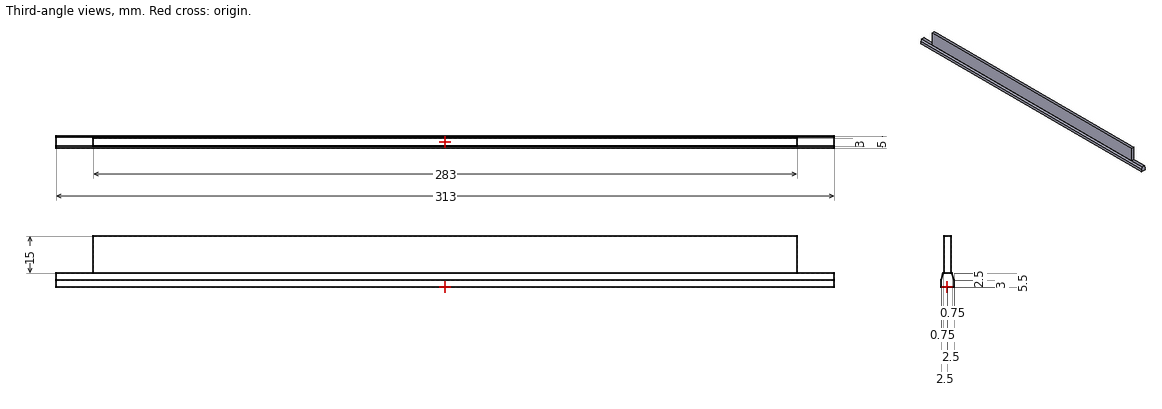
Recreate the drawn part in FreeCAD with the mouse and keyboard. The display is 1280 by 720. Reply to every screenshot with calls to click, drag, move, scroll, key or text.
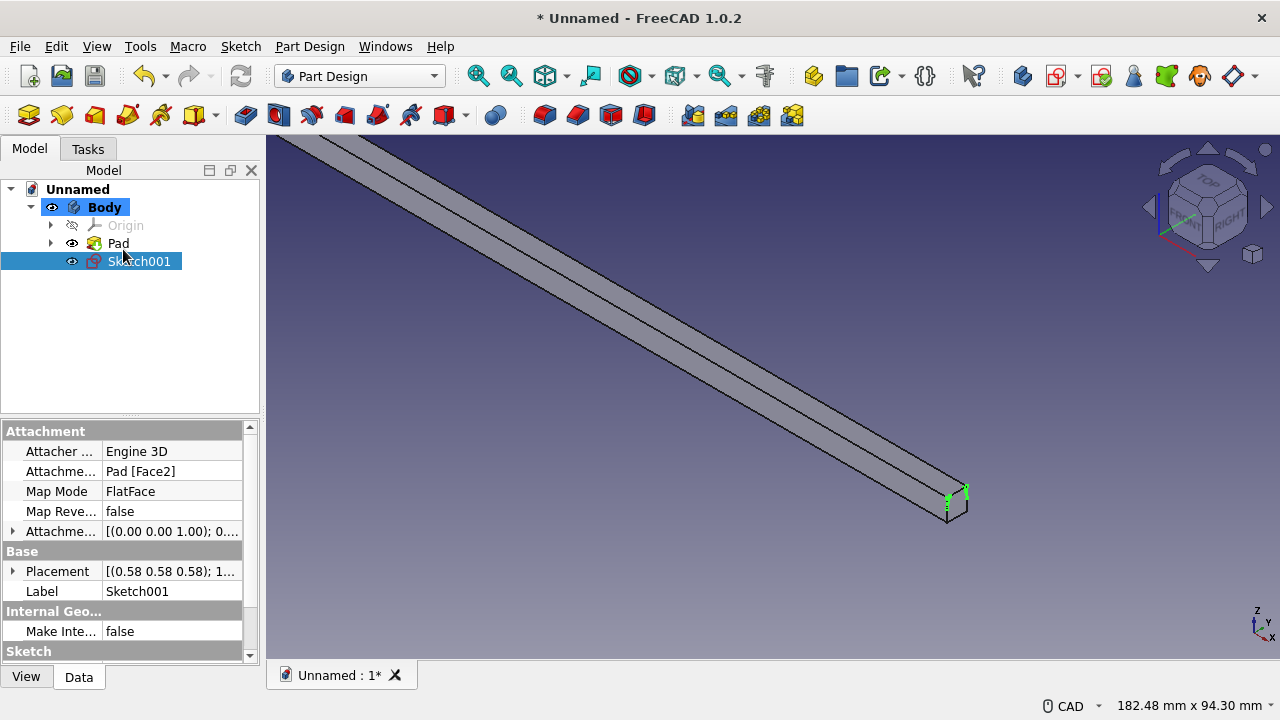
click(246, 116)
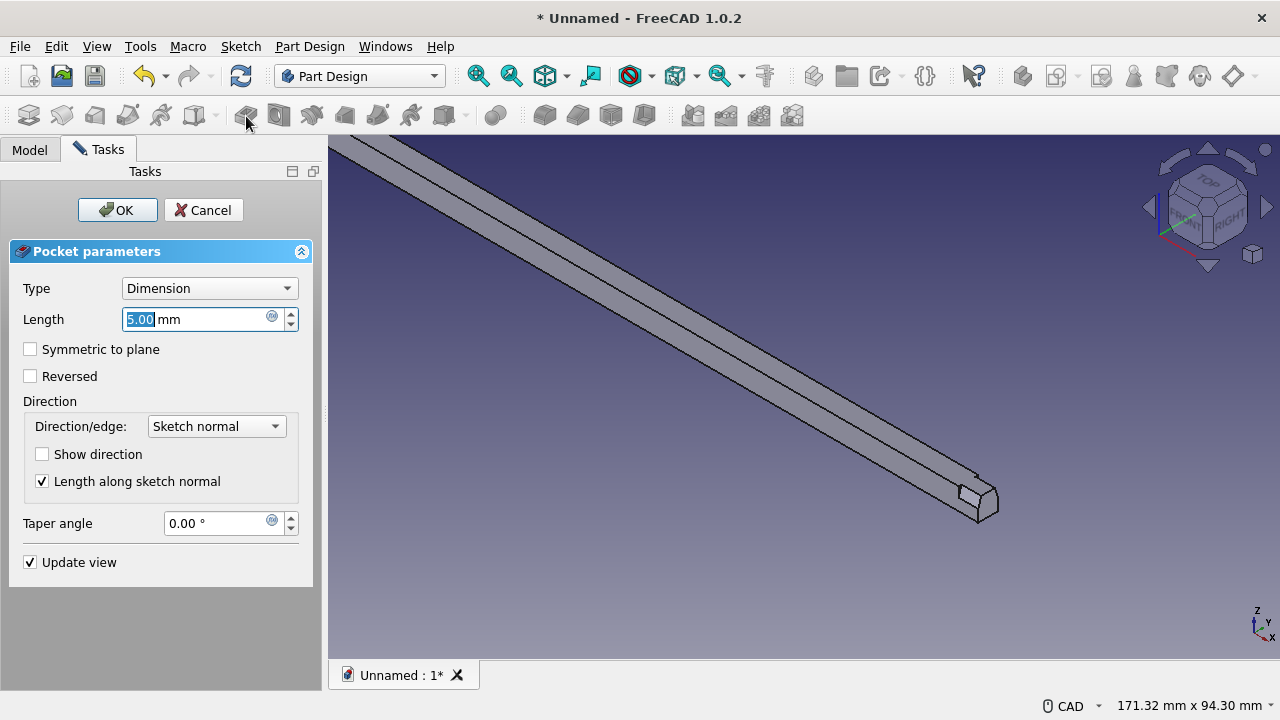
click(210, 288)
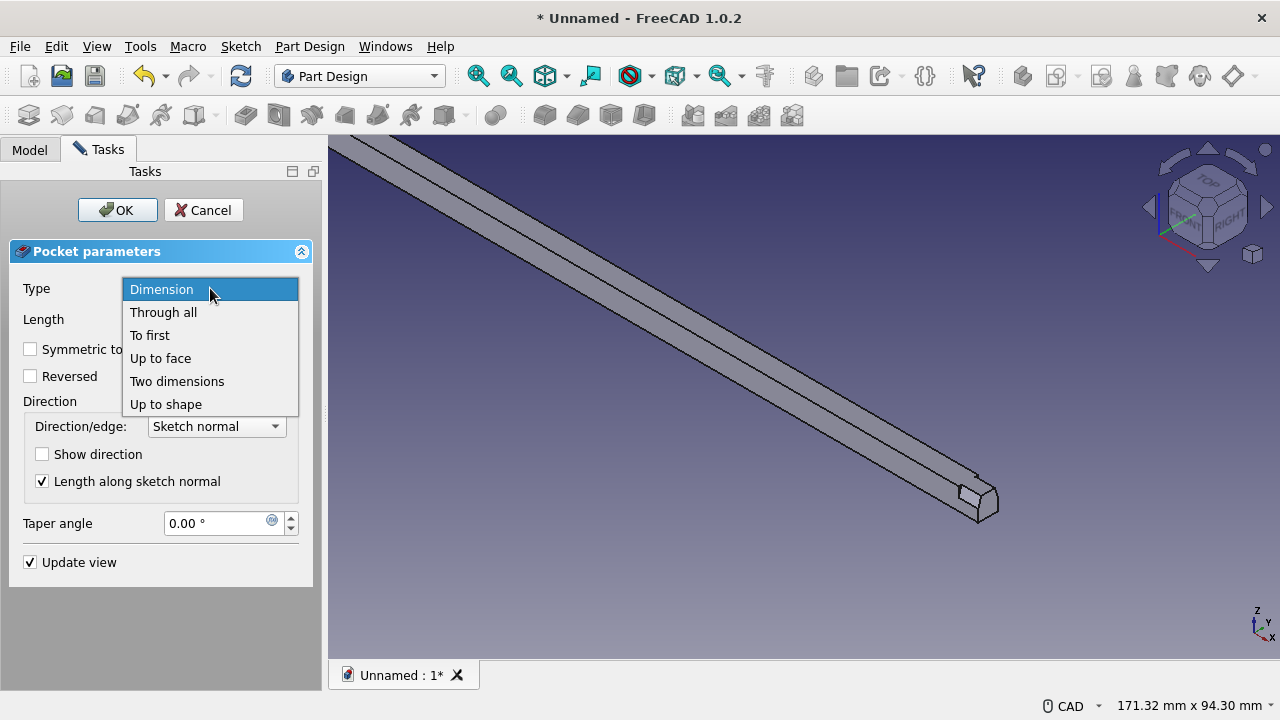
click(208, 312)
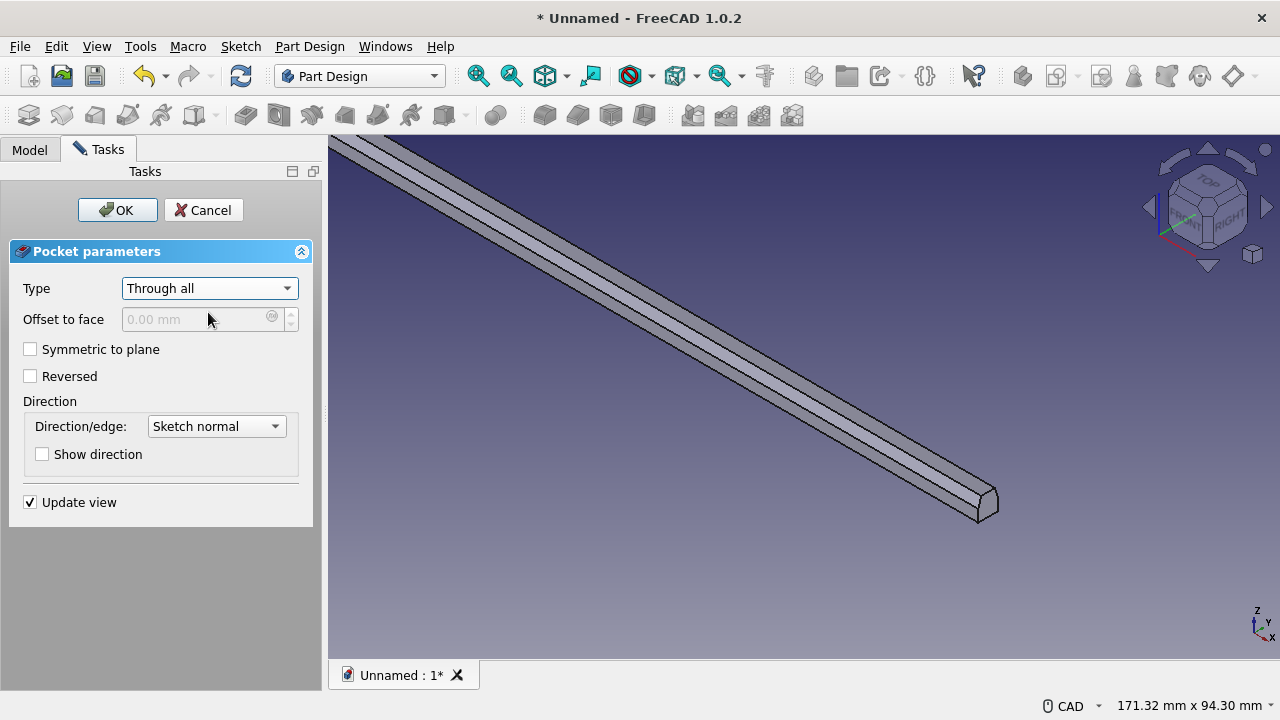
click(118, 210)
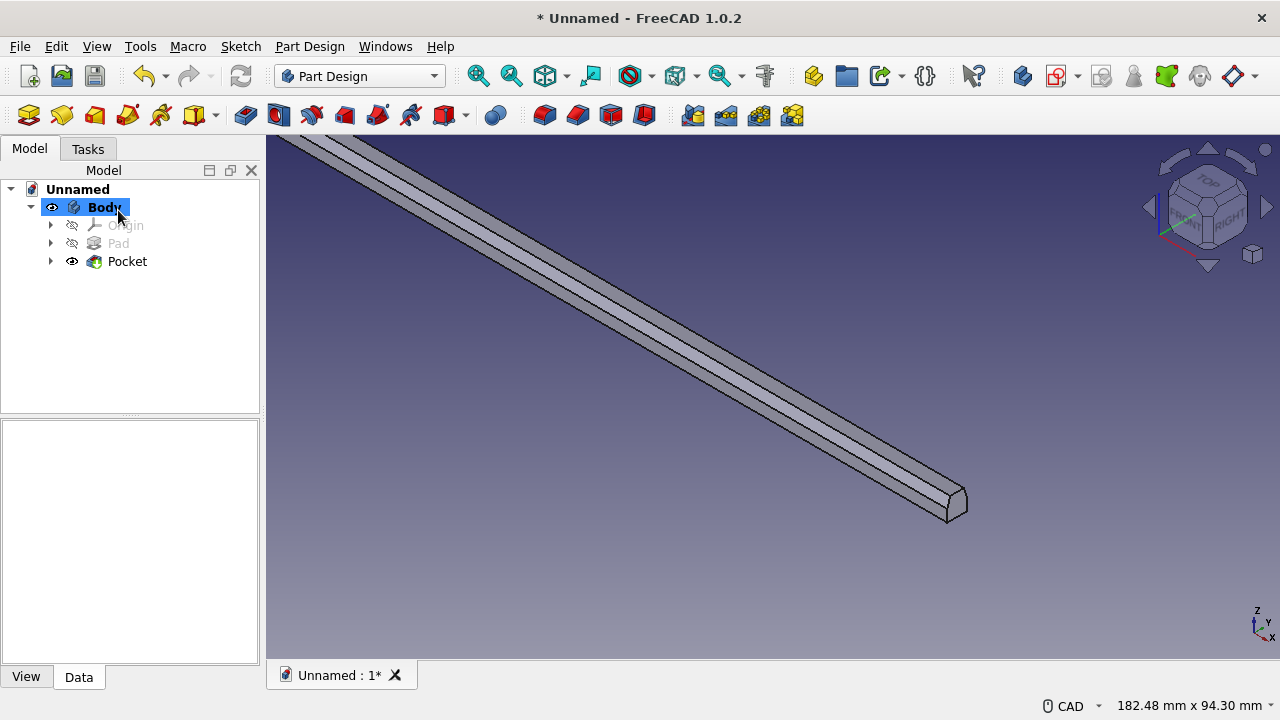
click(479, 76)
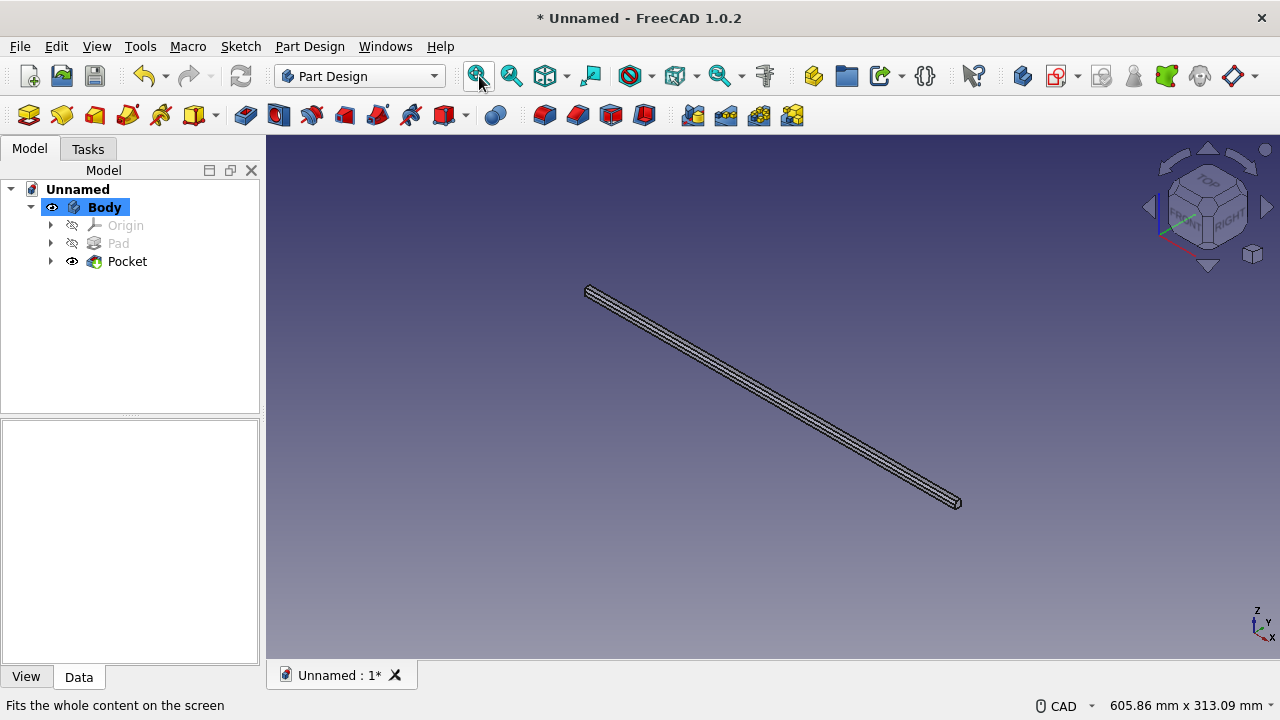
scroll(932, 484, up, 8)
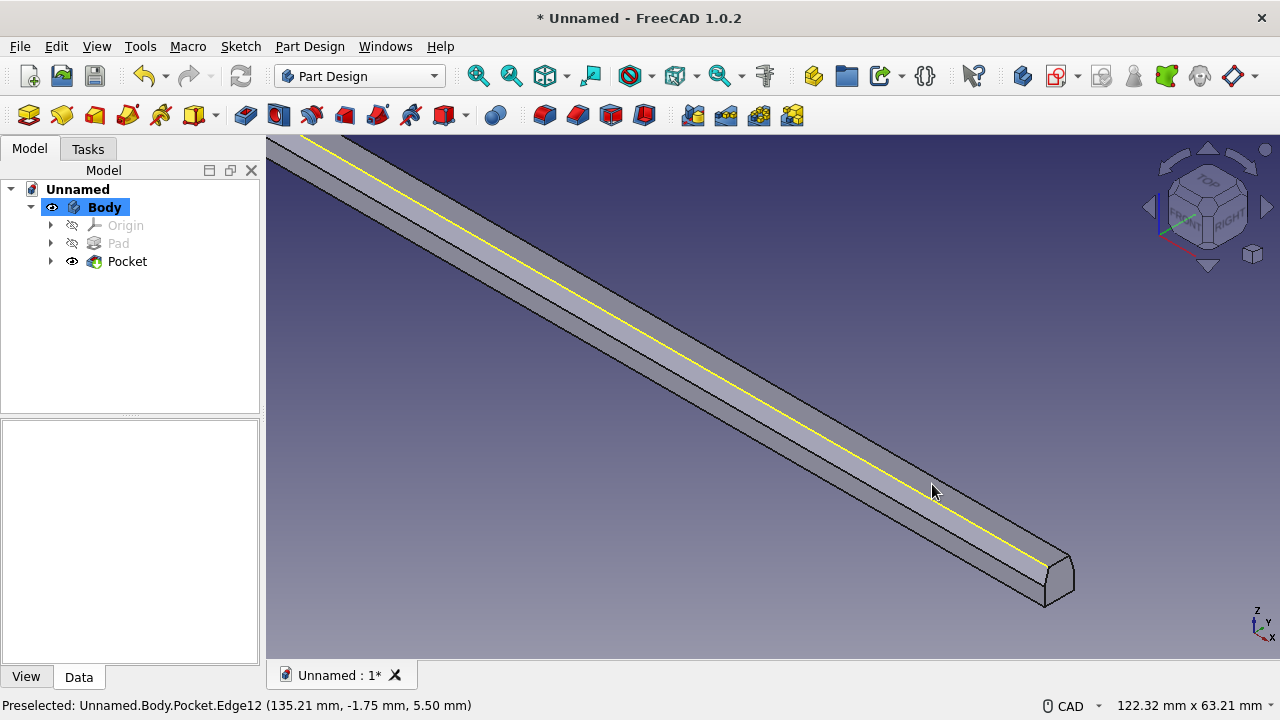
click(928, 485)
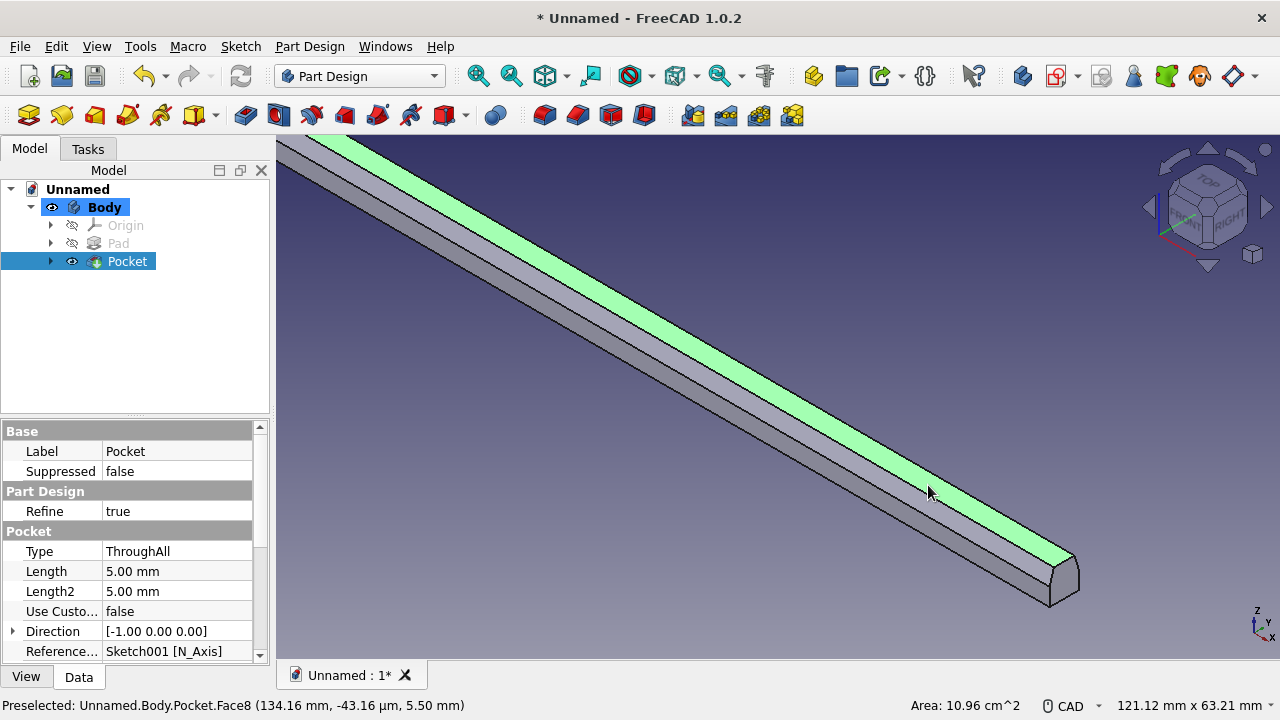
click(1056, 76)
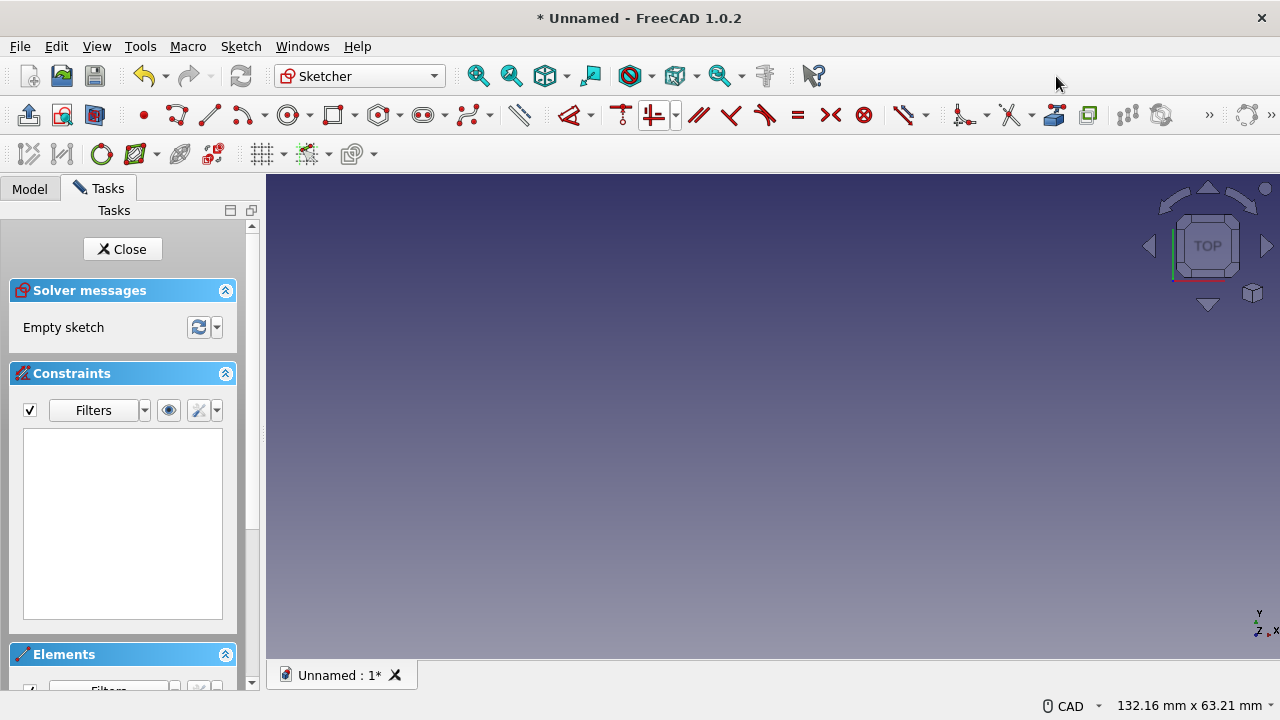
scroll(860, 324, down, 7)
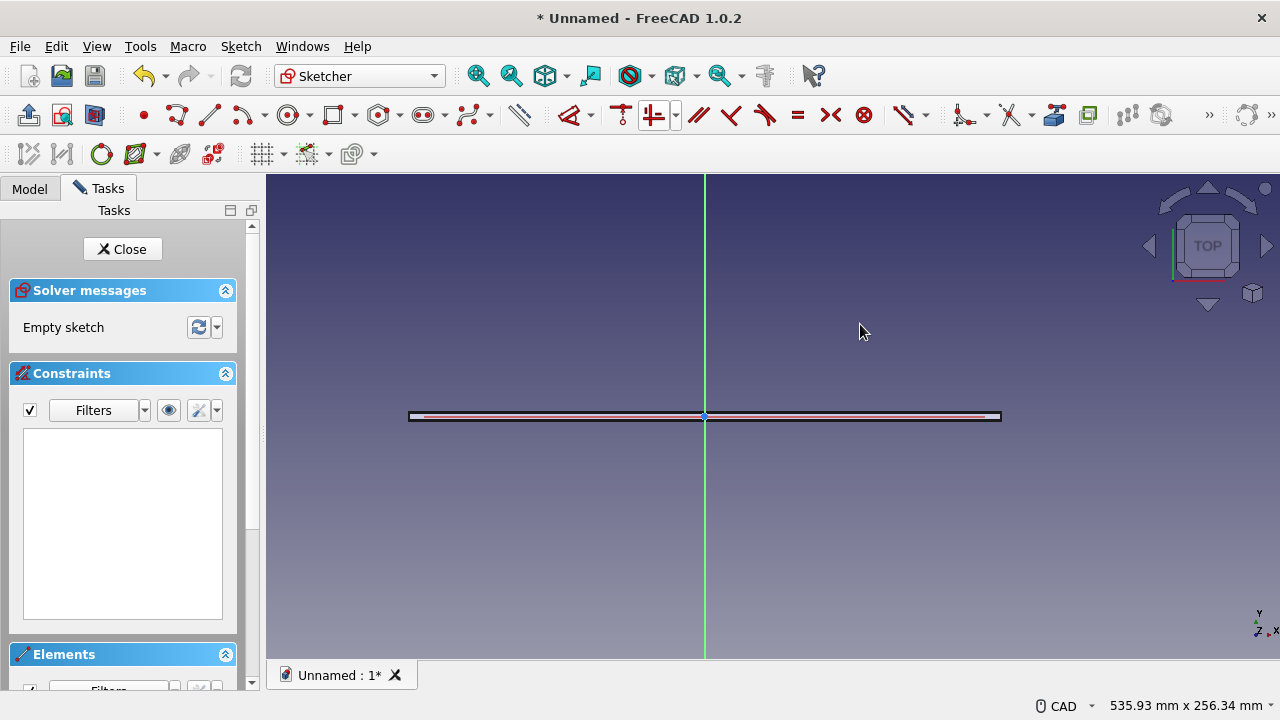
key(g)
key(v)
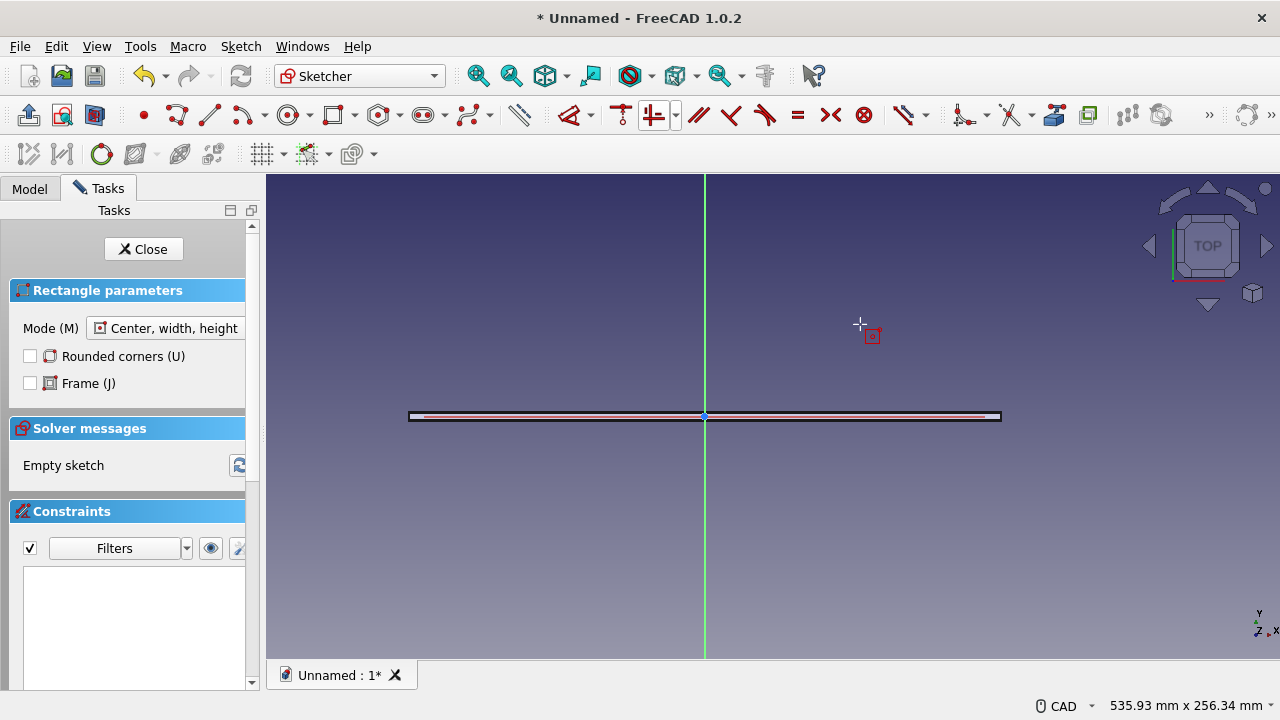
scroll(705, 417, up, 9)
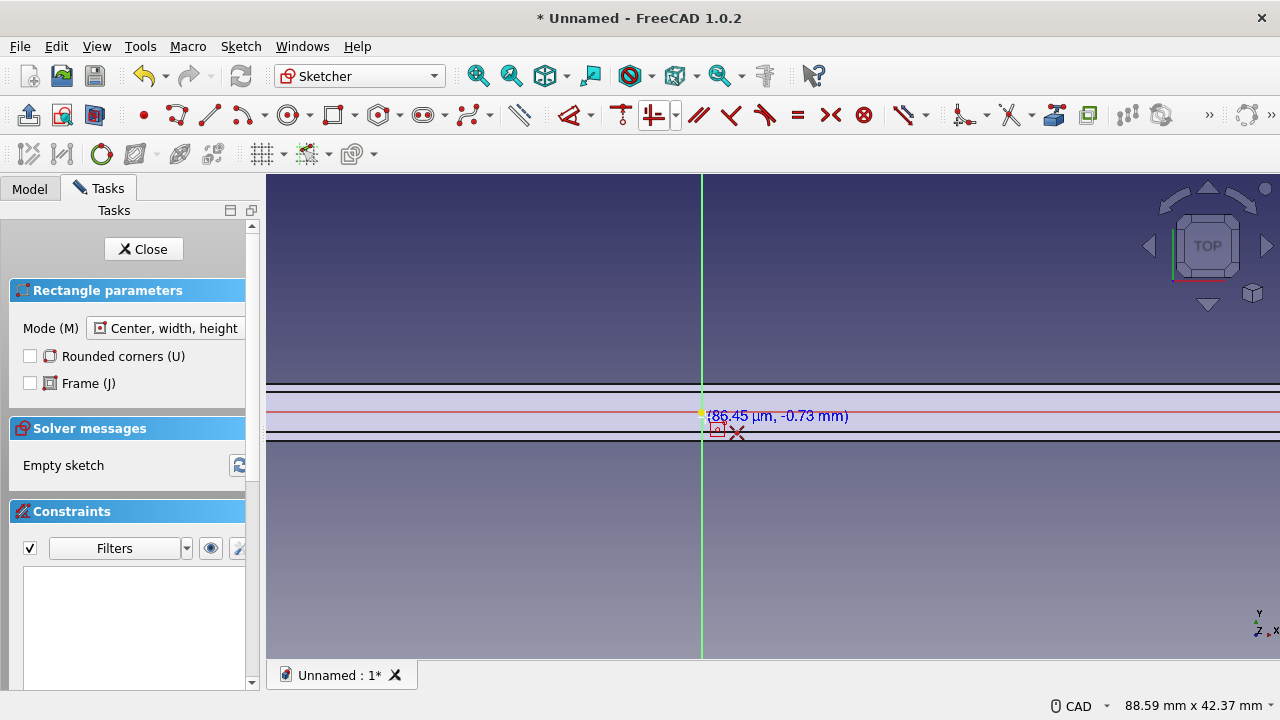
scroll(705, 417, down, 9)